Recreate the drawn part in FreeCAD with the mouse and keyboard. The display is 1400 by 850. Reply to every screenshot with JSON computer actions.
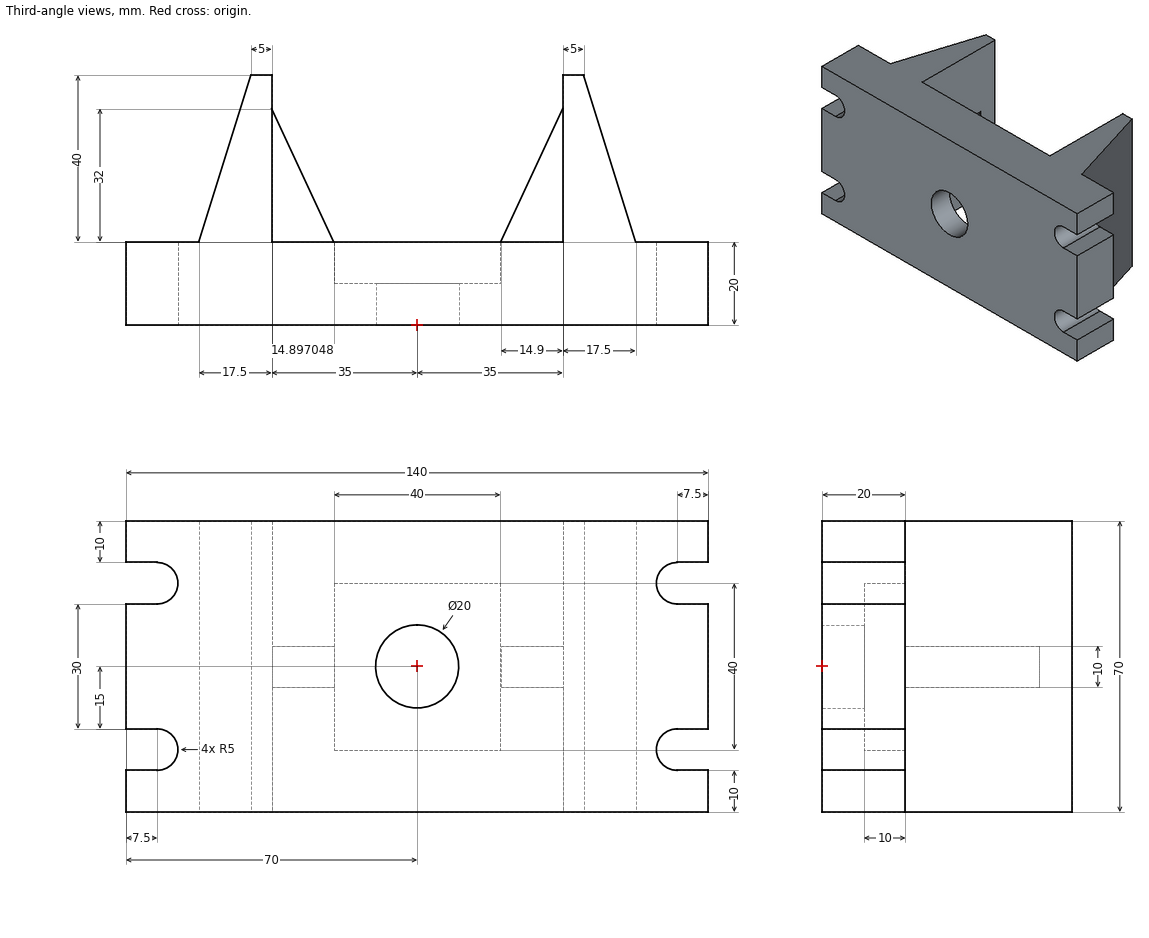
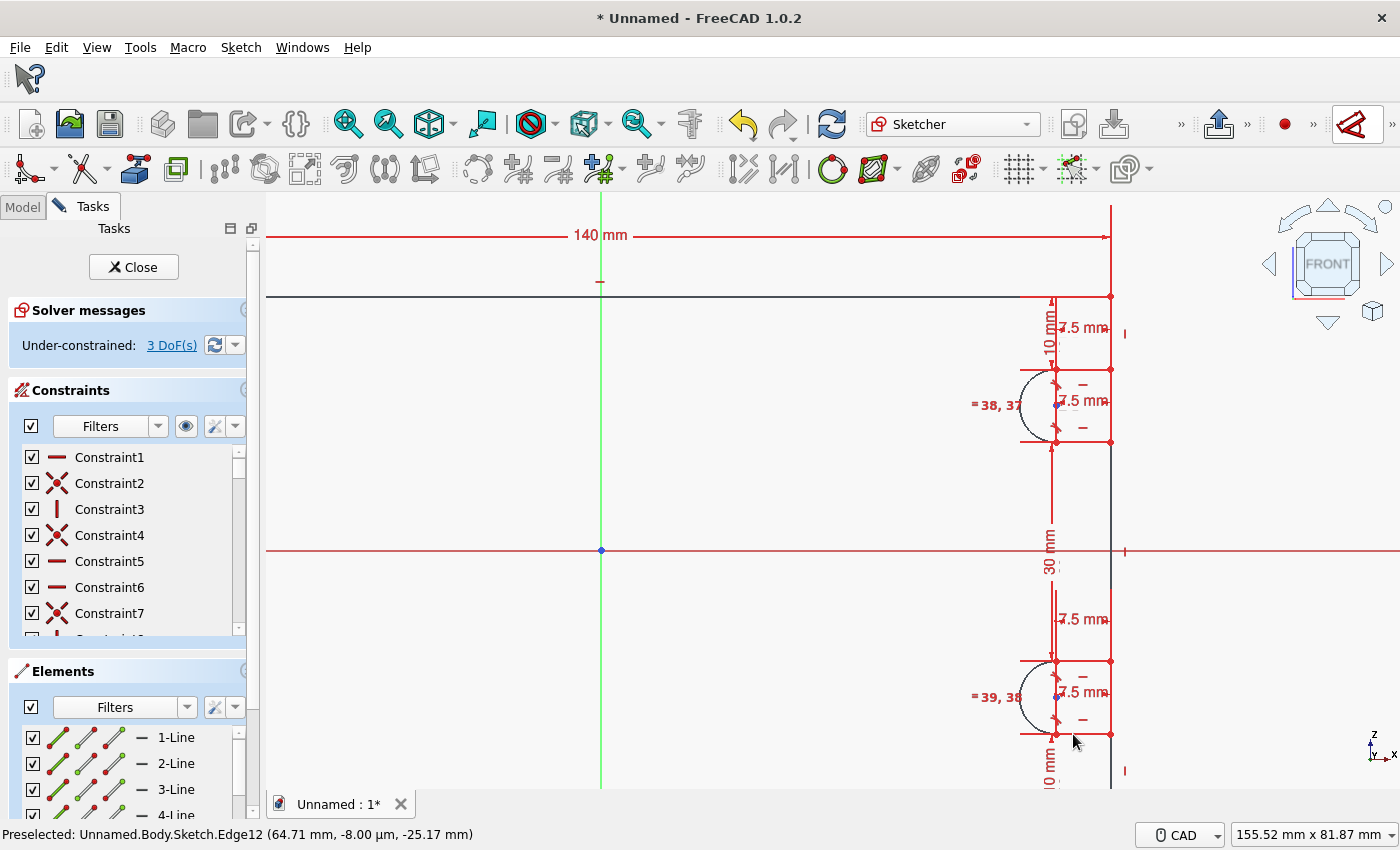
{"action": "scroll", "coordinate": [1097, 368], "scroll_direction": "down", "scroll_amount": 2}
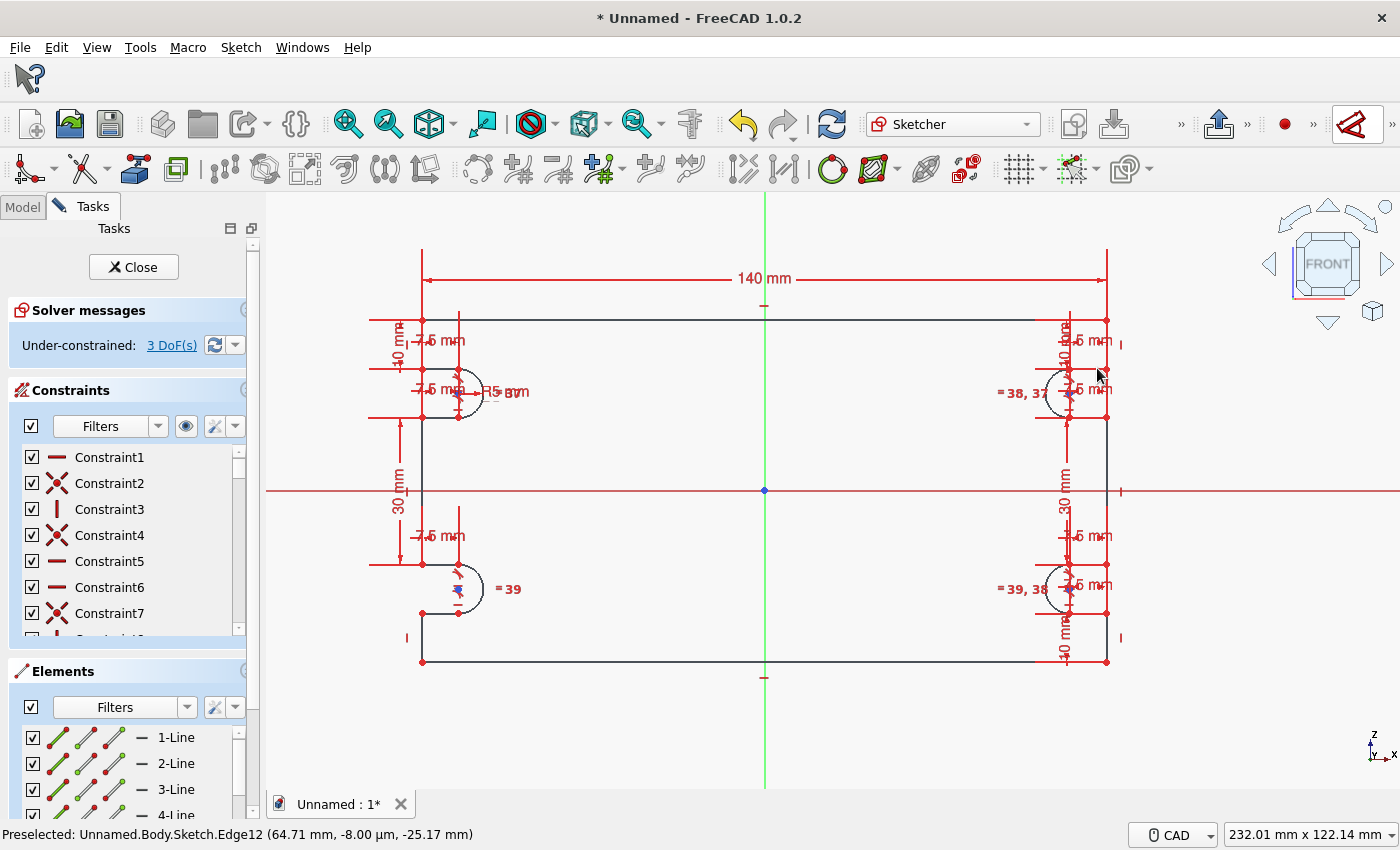
{"action": "left_click", "coordinate": [901, 662]}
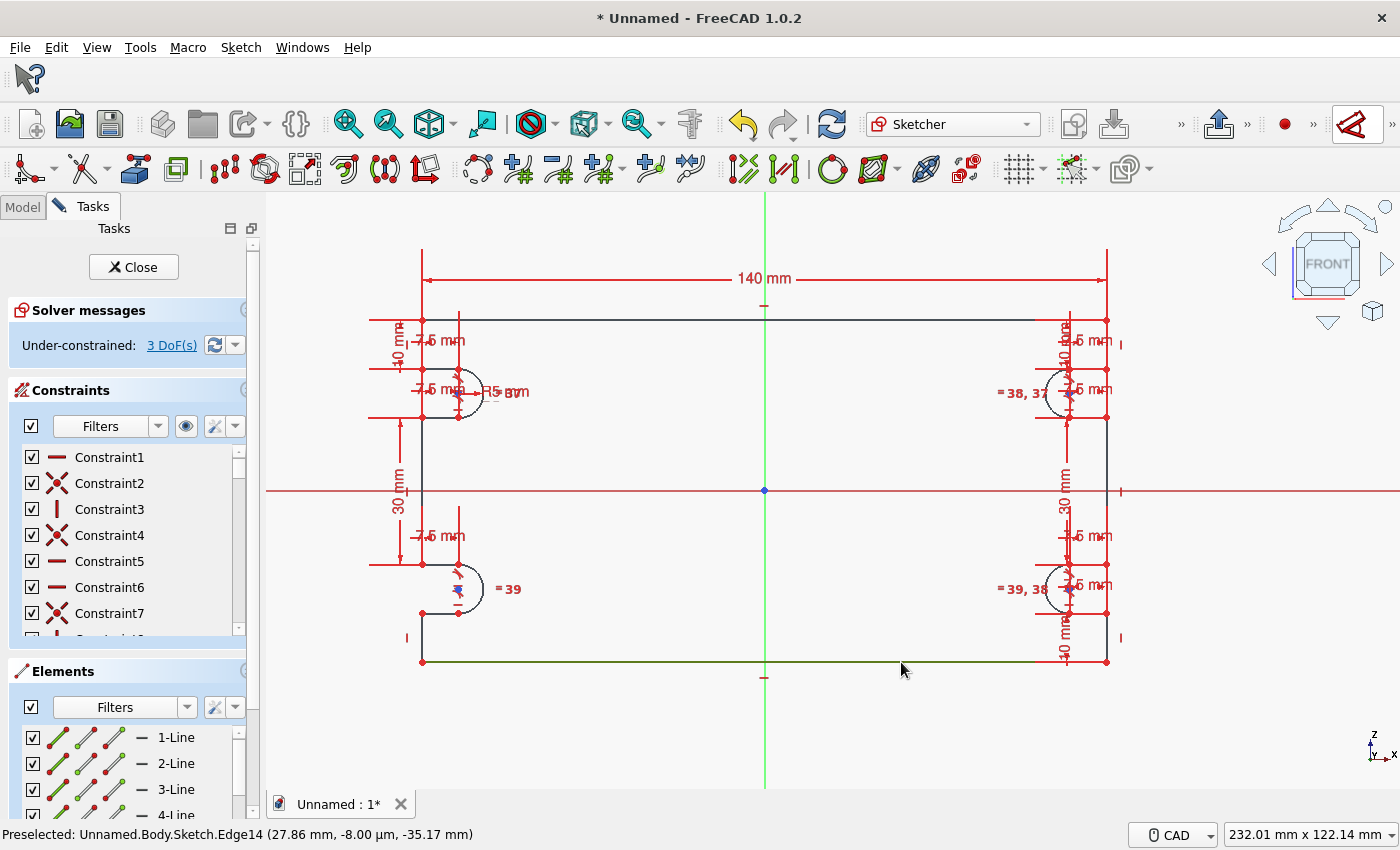
{"action": "key", "text": "l"}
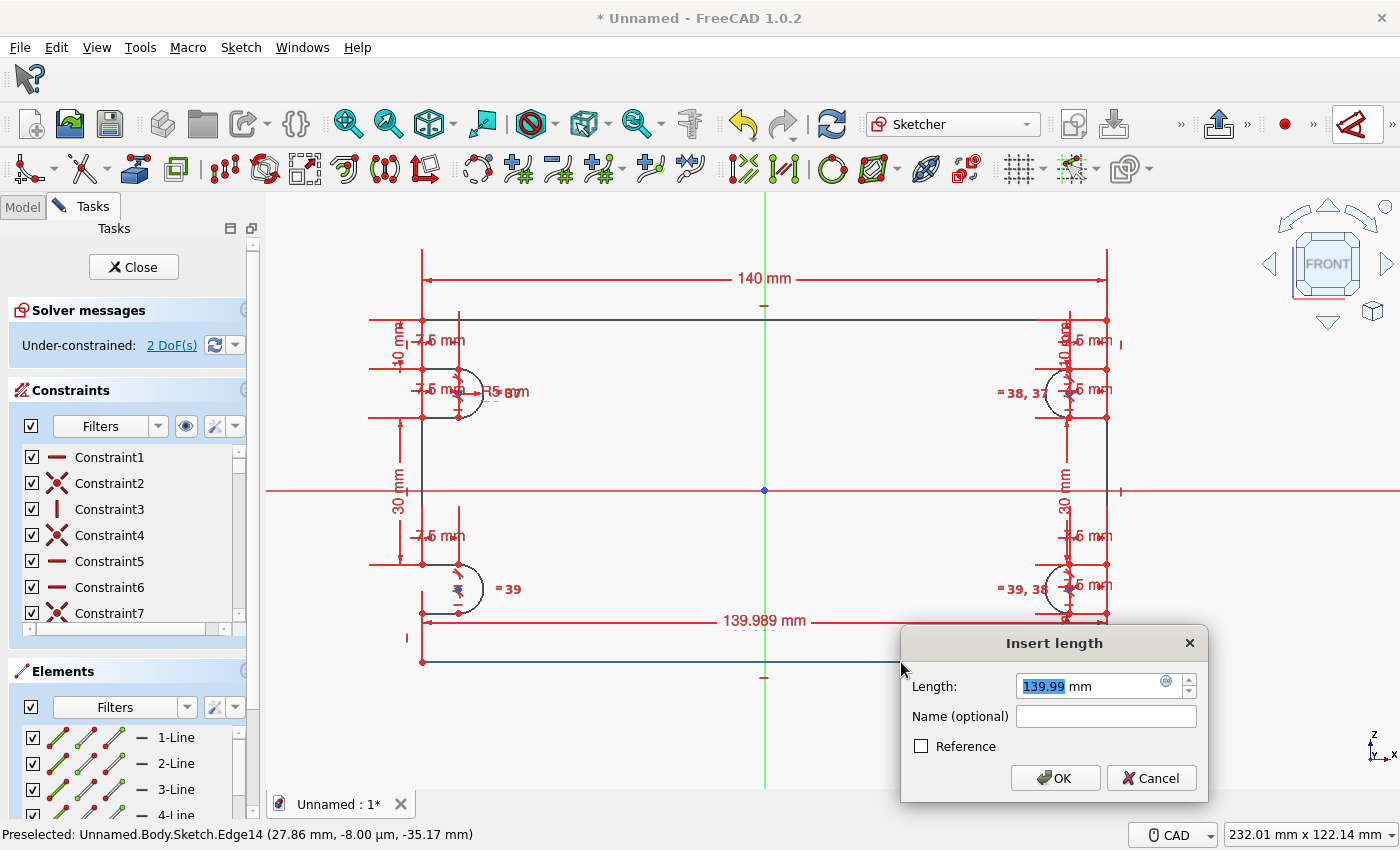
{"action": "type", "text": "140"}
{"action": "key", "text": "Return"}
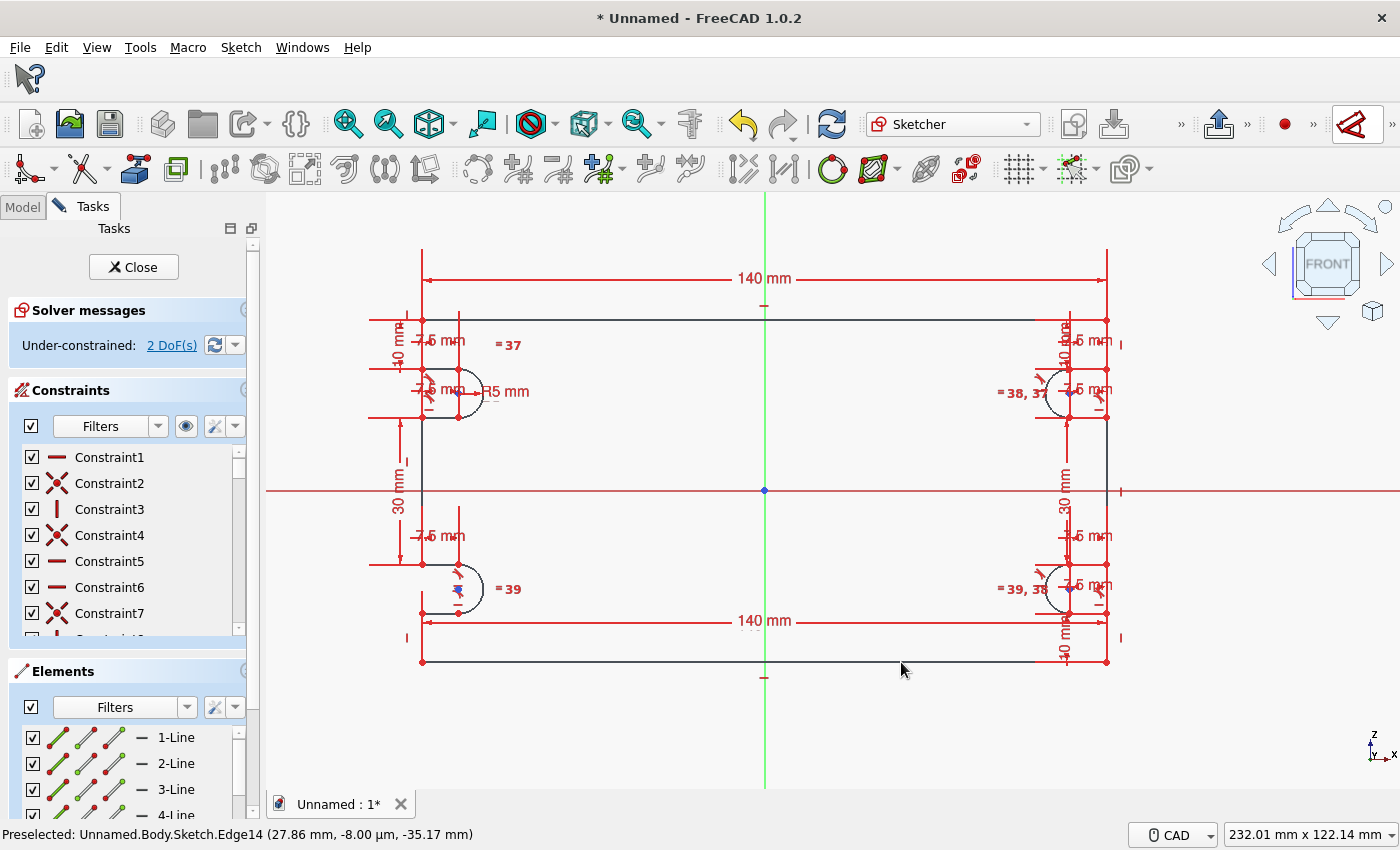
{"action": "left_click", "coordinate": [459, 565]}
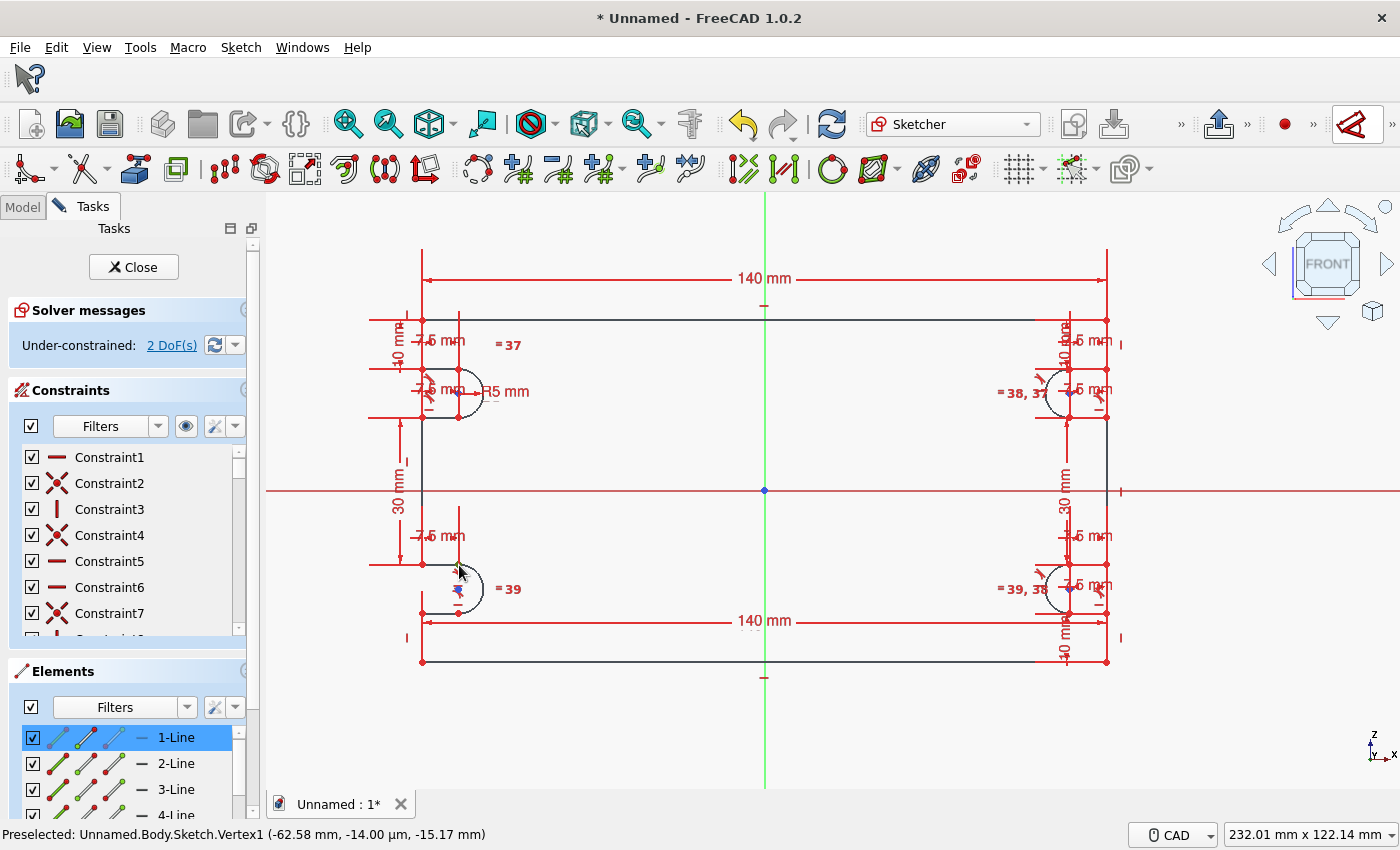
{"action": "left_click", "coordinate": [1378, 124]}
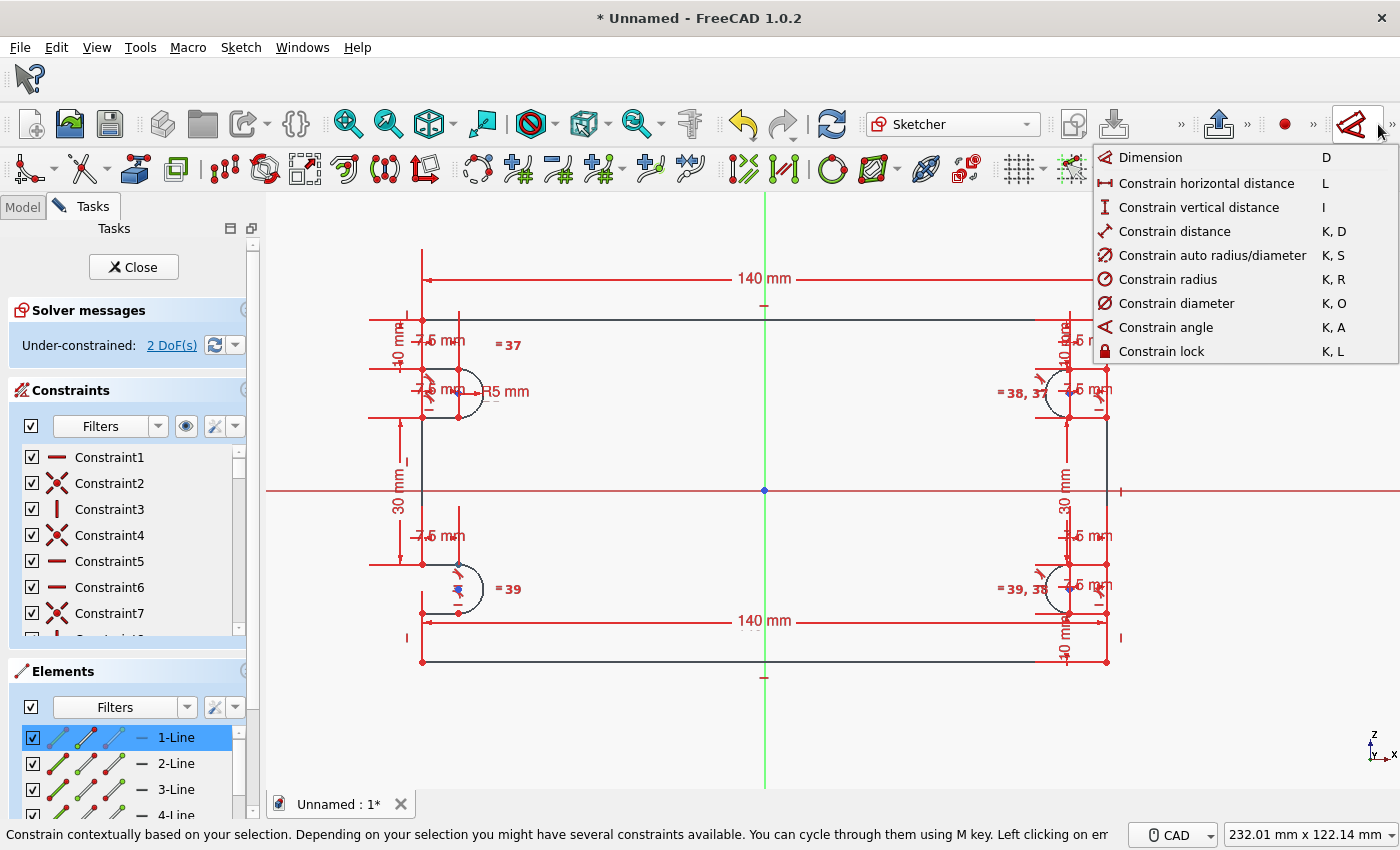
{"action": "left_click", "coordinate": [1246, 207]}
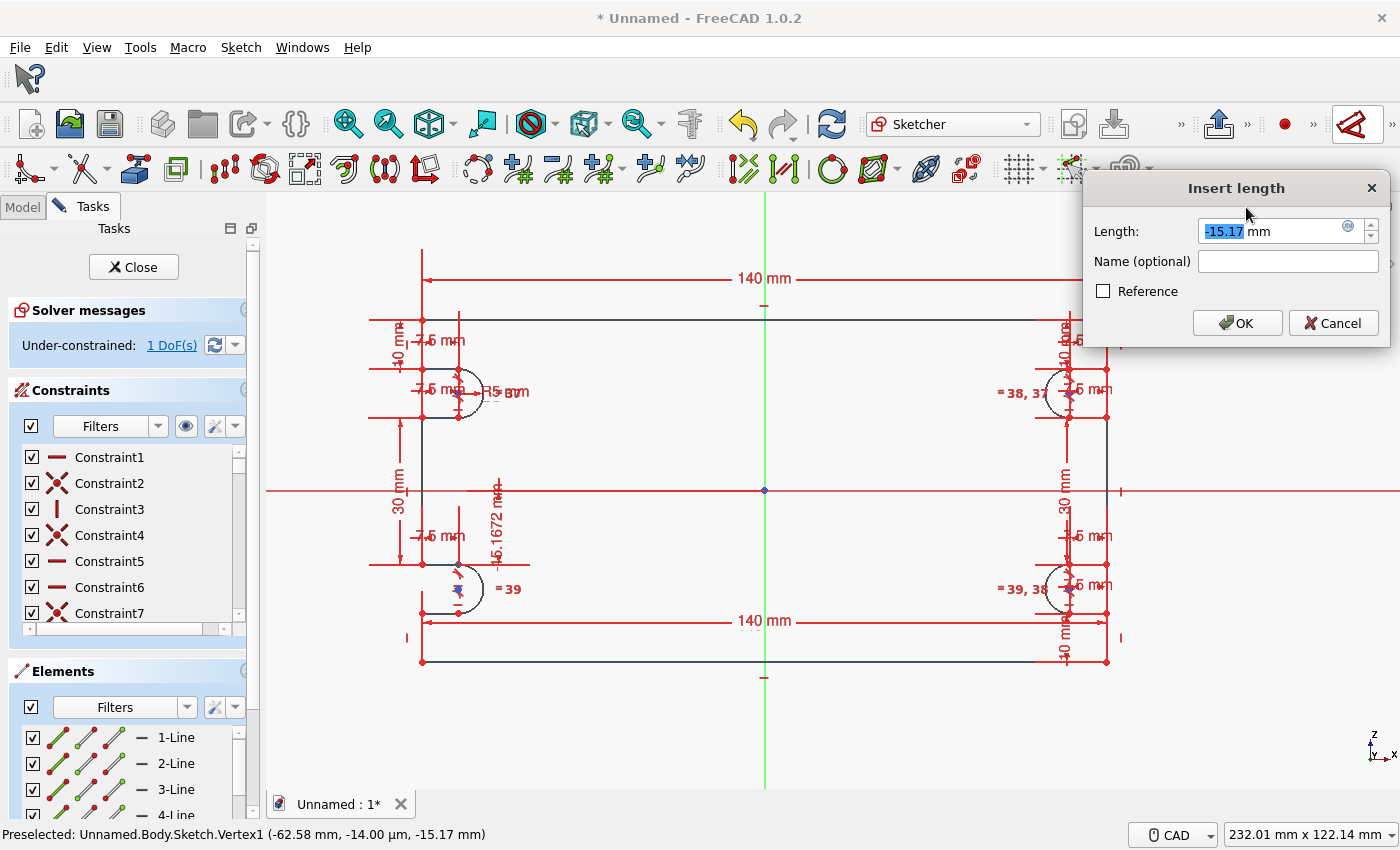
{"action": "type", "text": "-15"}
{"action": "key", "text": "Return"}